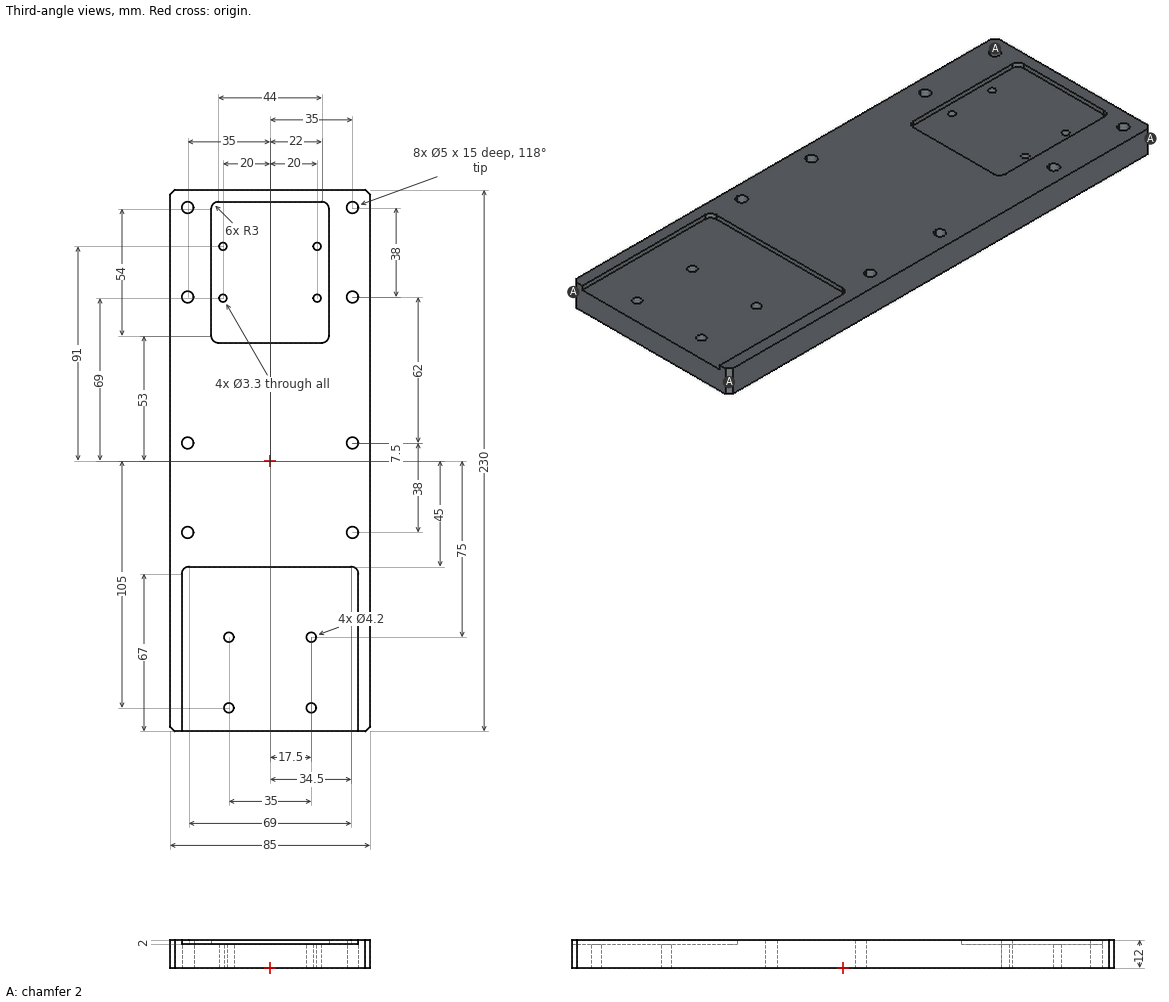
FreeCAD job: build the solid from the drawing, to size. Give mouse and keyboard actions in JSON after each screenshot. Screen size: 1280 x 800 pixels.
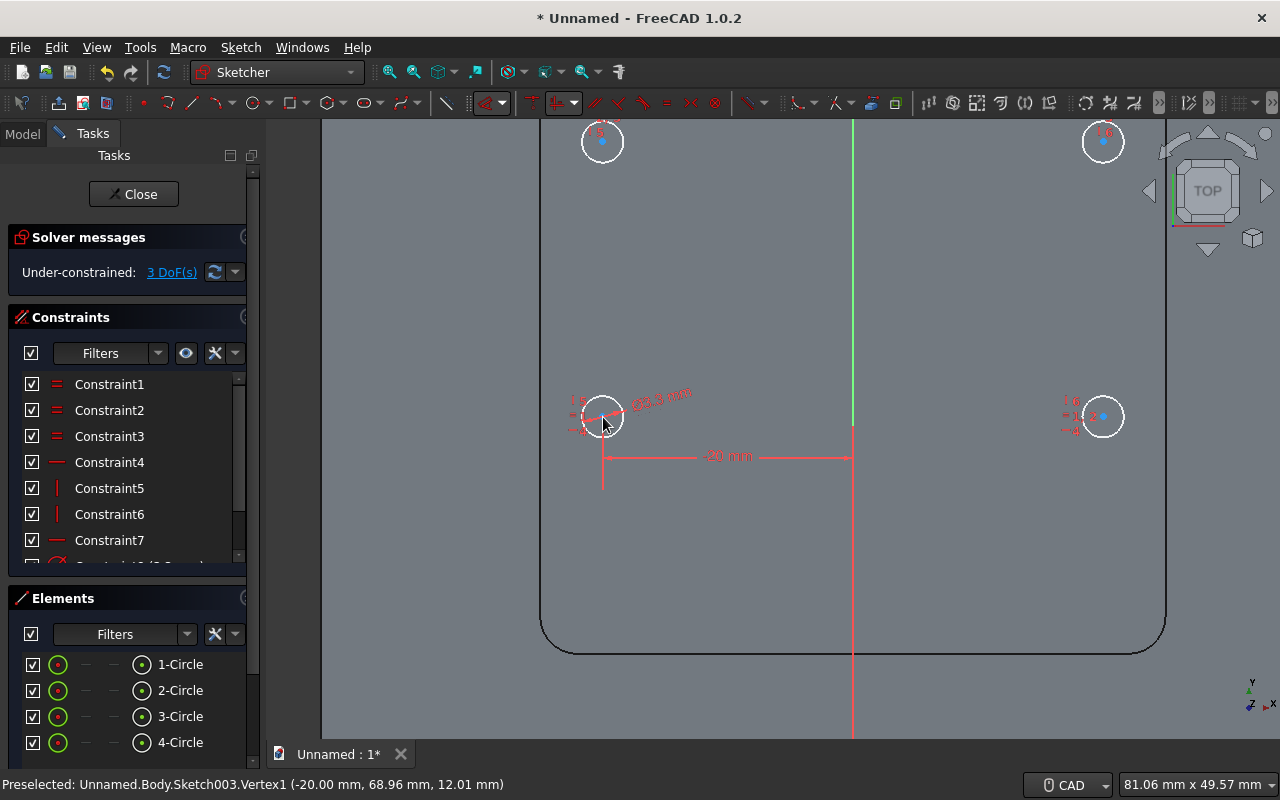
{"action": "left_click", "coordinate": [603, 417]}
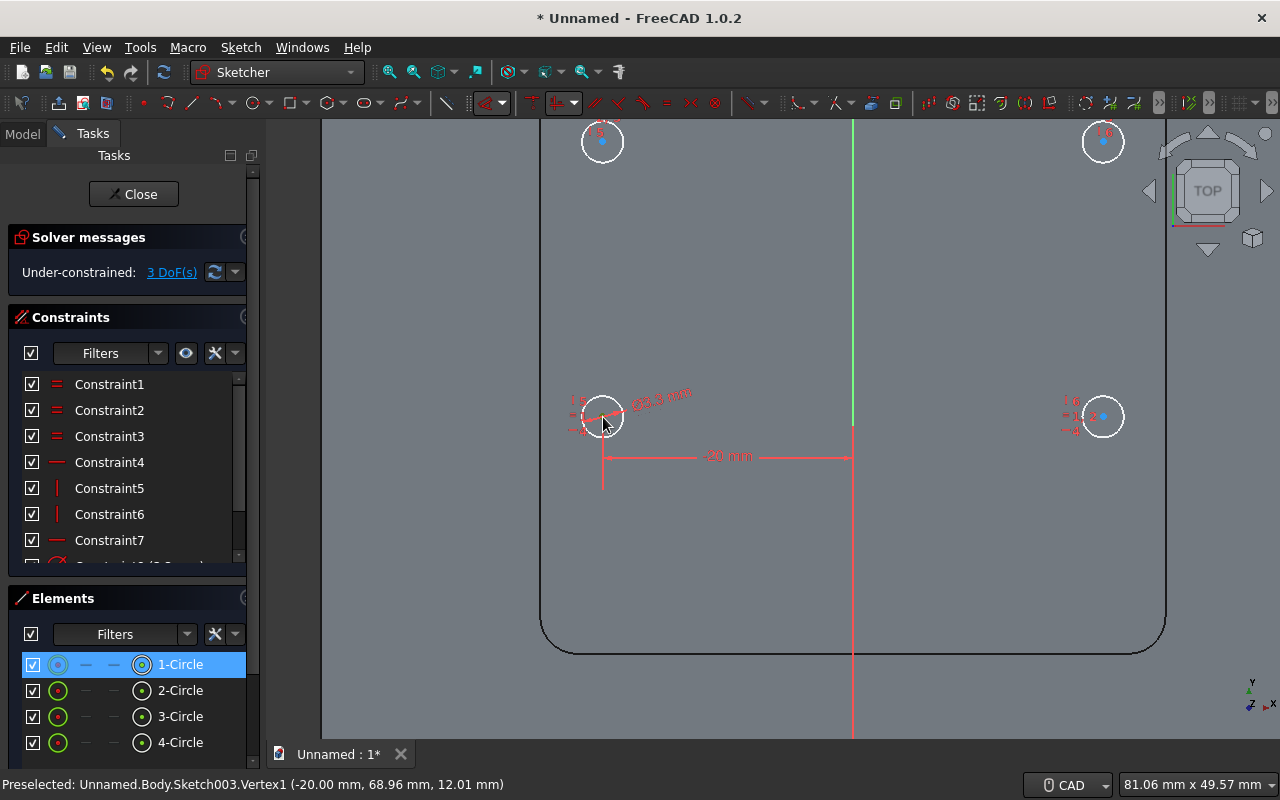
{"action": "key", "text": "i"}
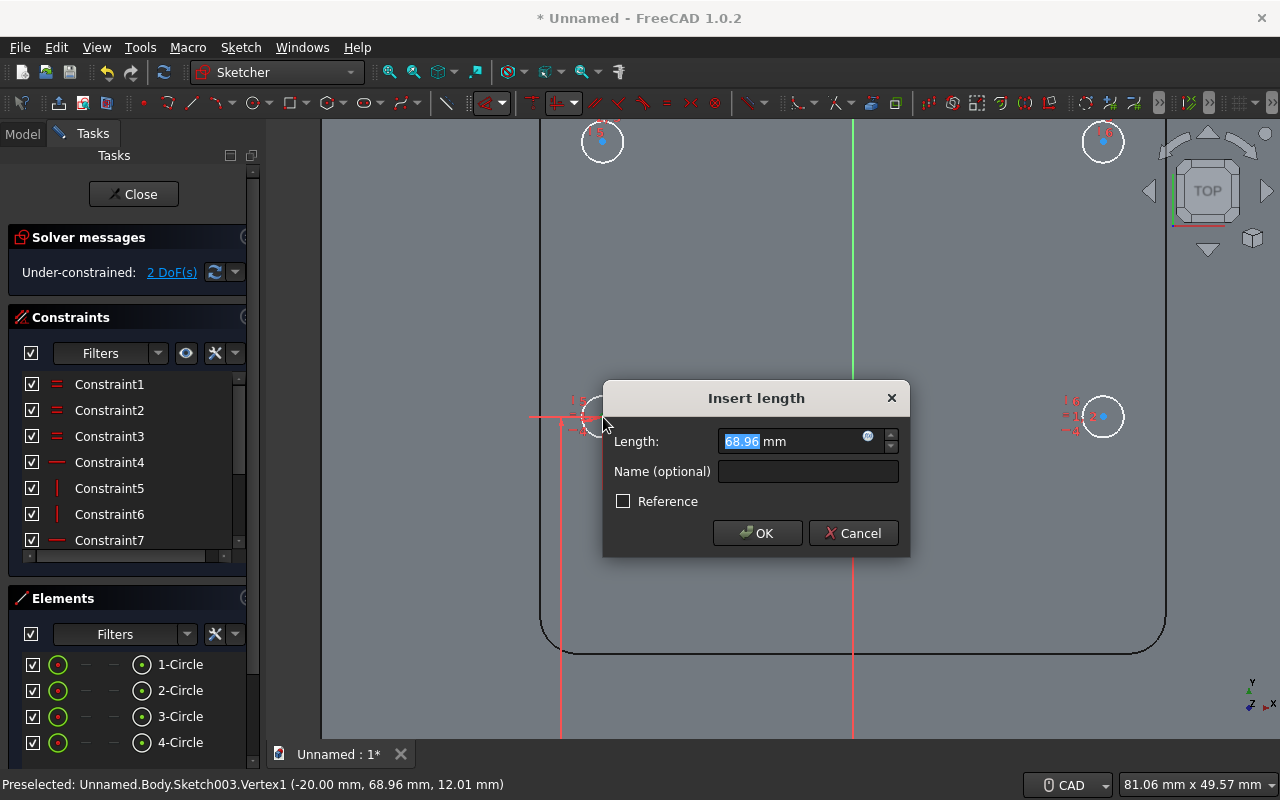
{"action": "type", "text": "69"}
{"action": "key", "text": "Return"}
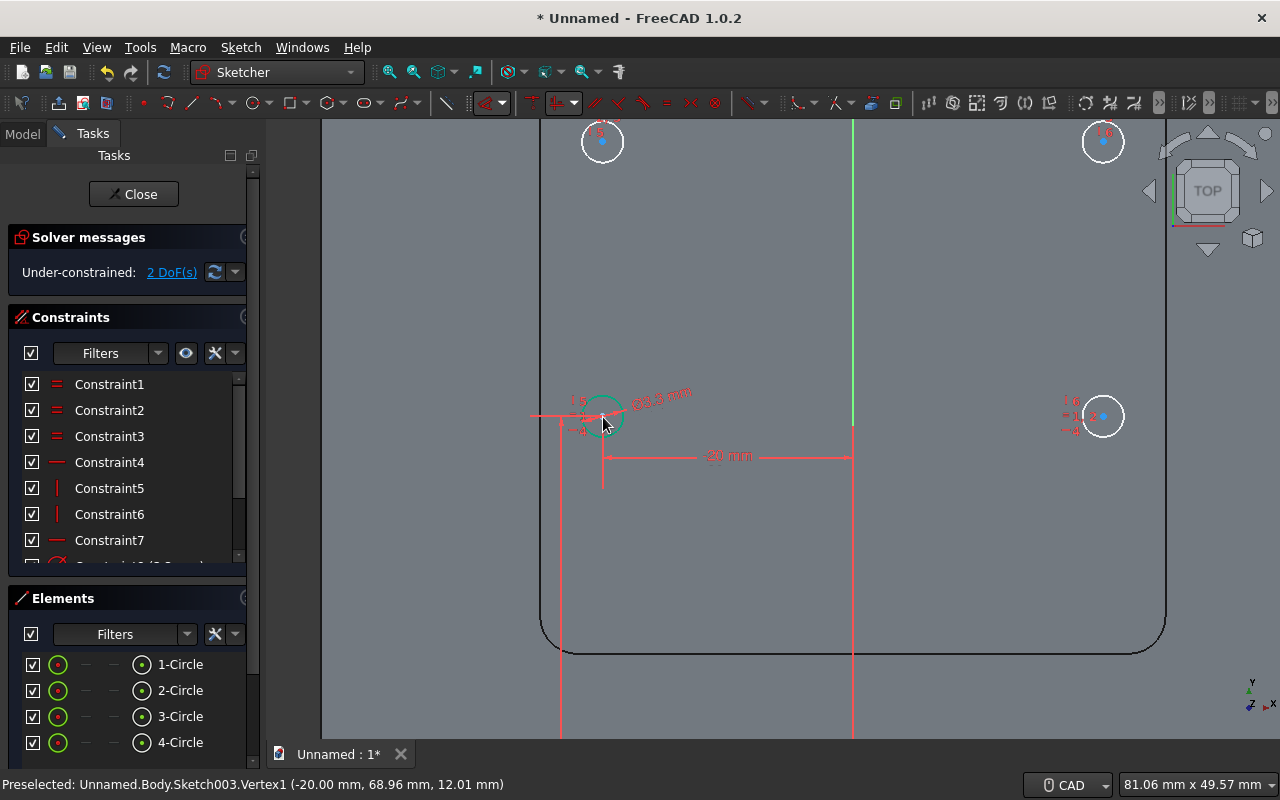
{"action": "left_click", "coordinate": [1103, 416]}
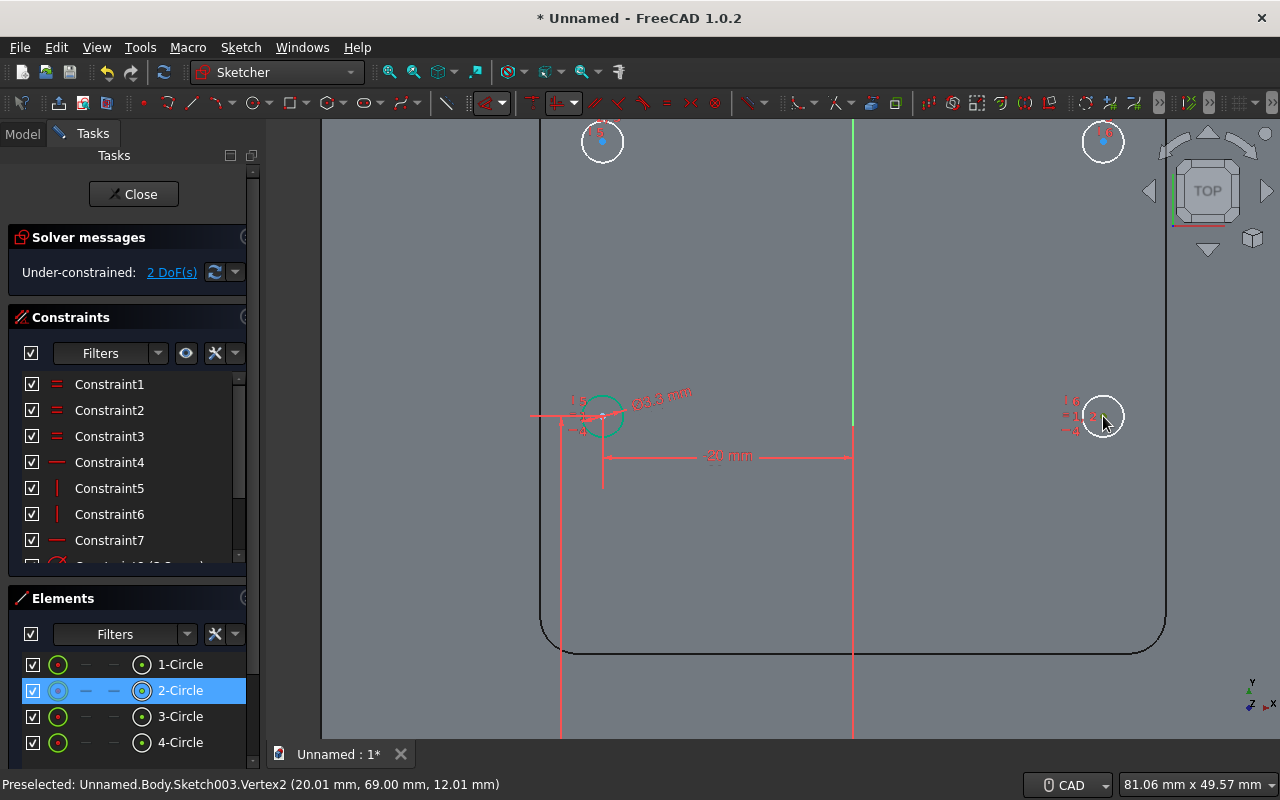
{"action": "key", "text": "l"}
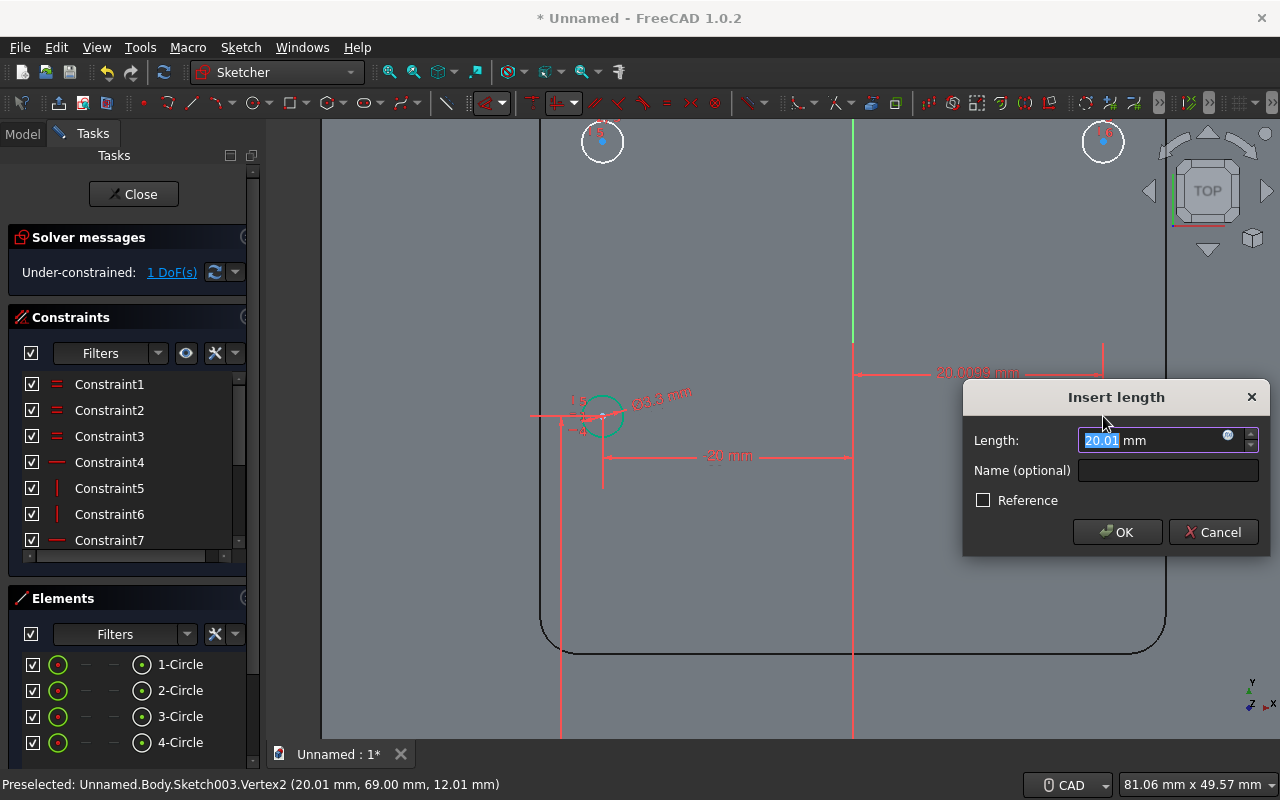
{"action": "type", "text": "20"}
{"action": "key", "text": "Return"}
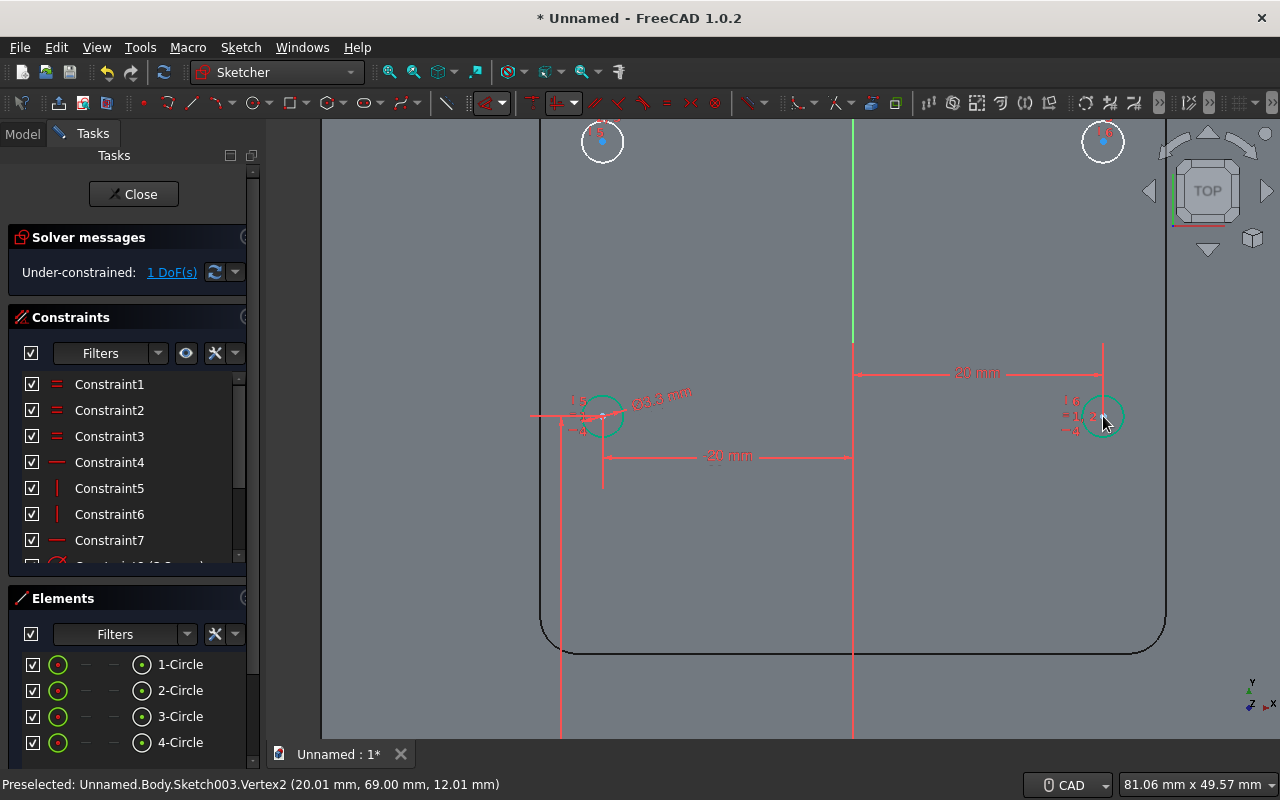
{"action": "scroll", "coordinate": [618, 271], "scroll_direction": "down", "scroll_amount": 5}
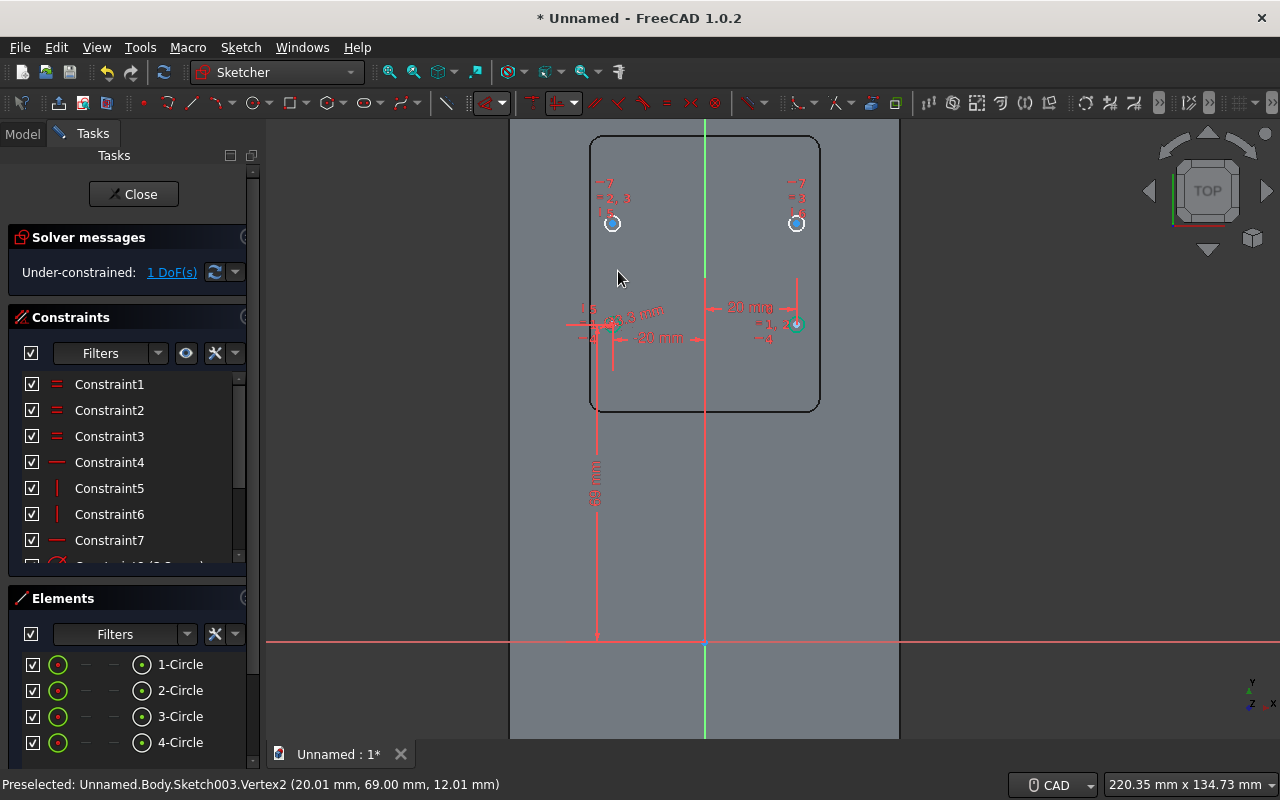
{"action": "left_click", "coordinate": [613, 224]}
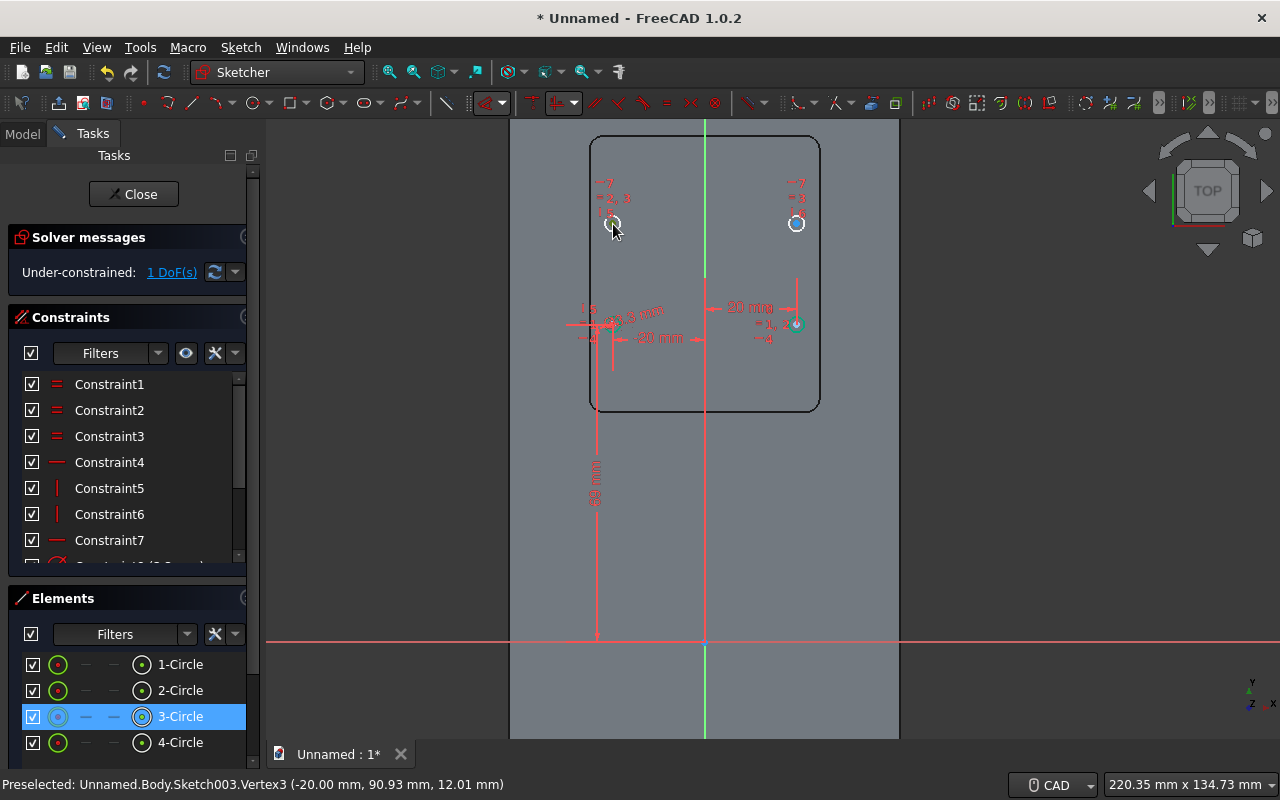
{"action": "key", "text": "i"}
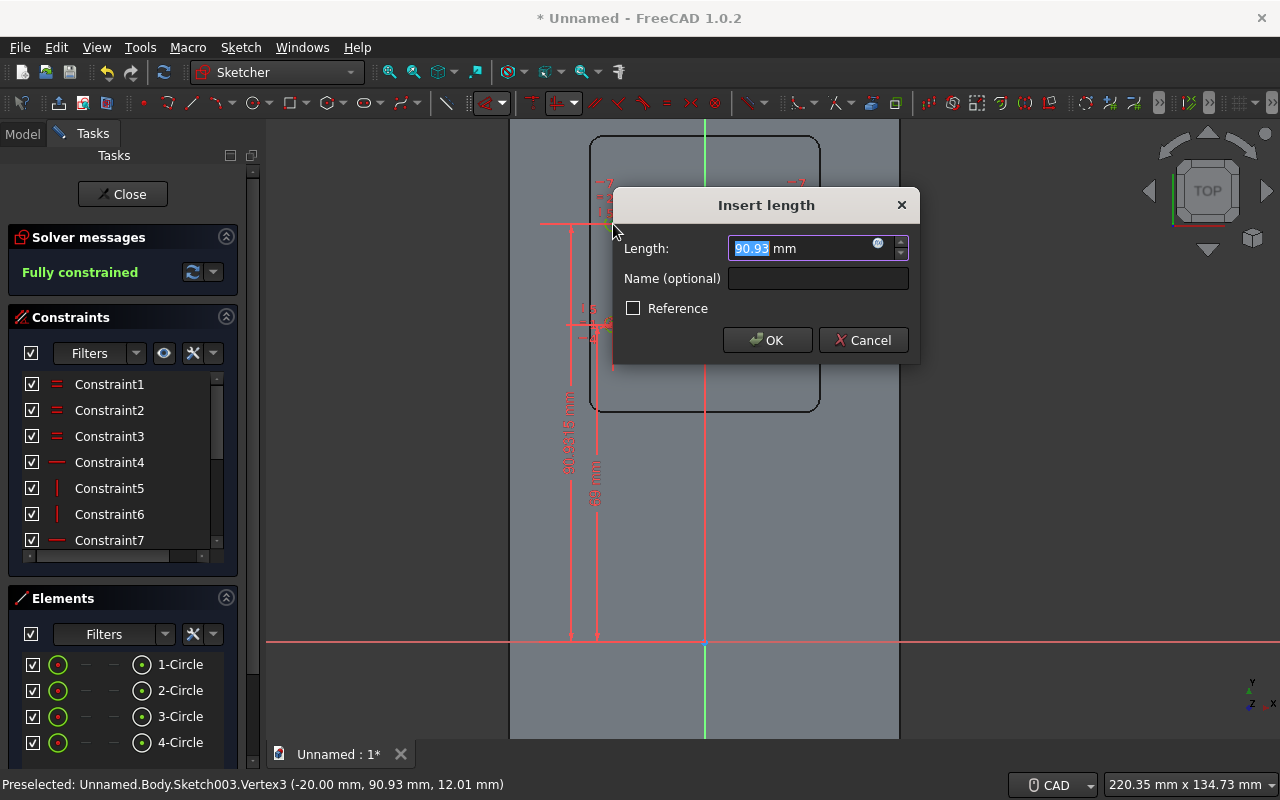
{"action": "type", "text": "91"}
{"action": "key", "text": "Return"}